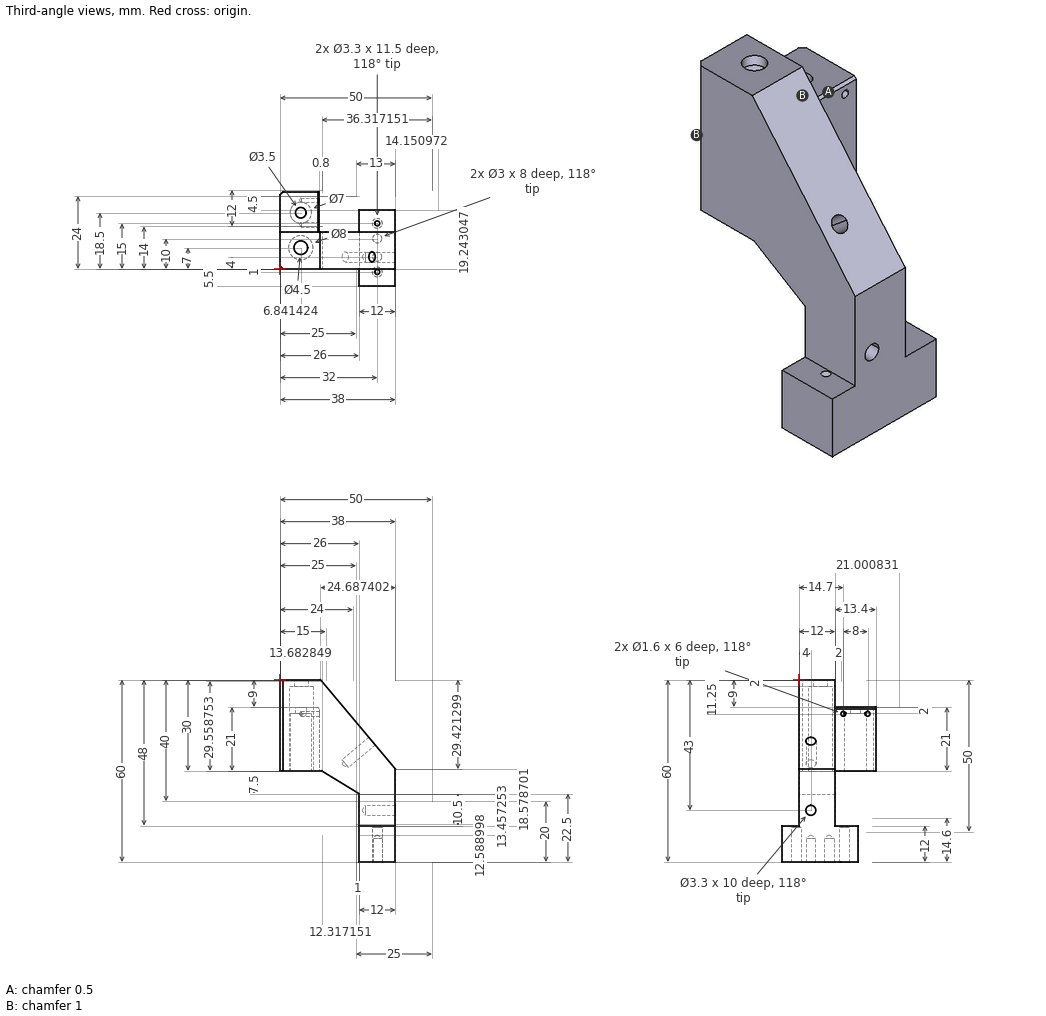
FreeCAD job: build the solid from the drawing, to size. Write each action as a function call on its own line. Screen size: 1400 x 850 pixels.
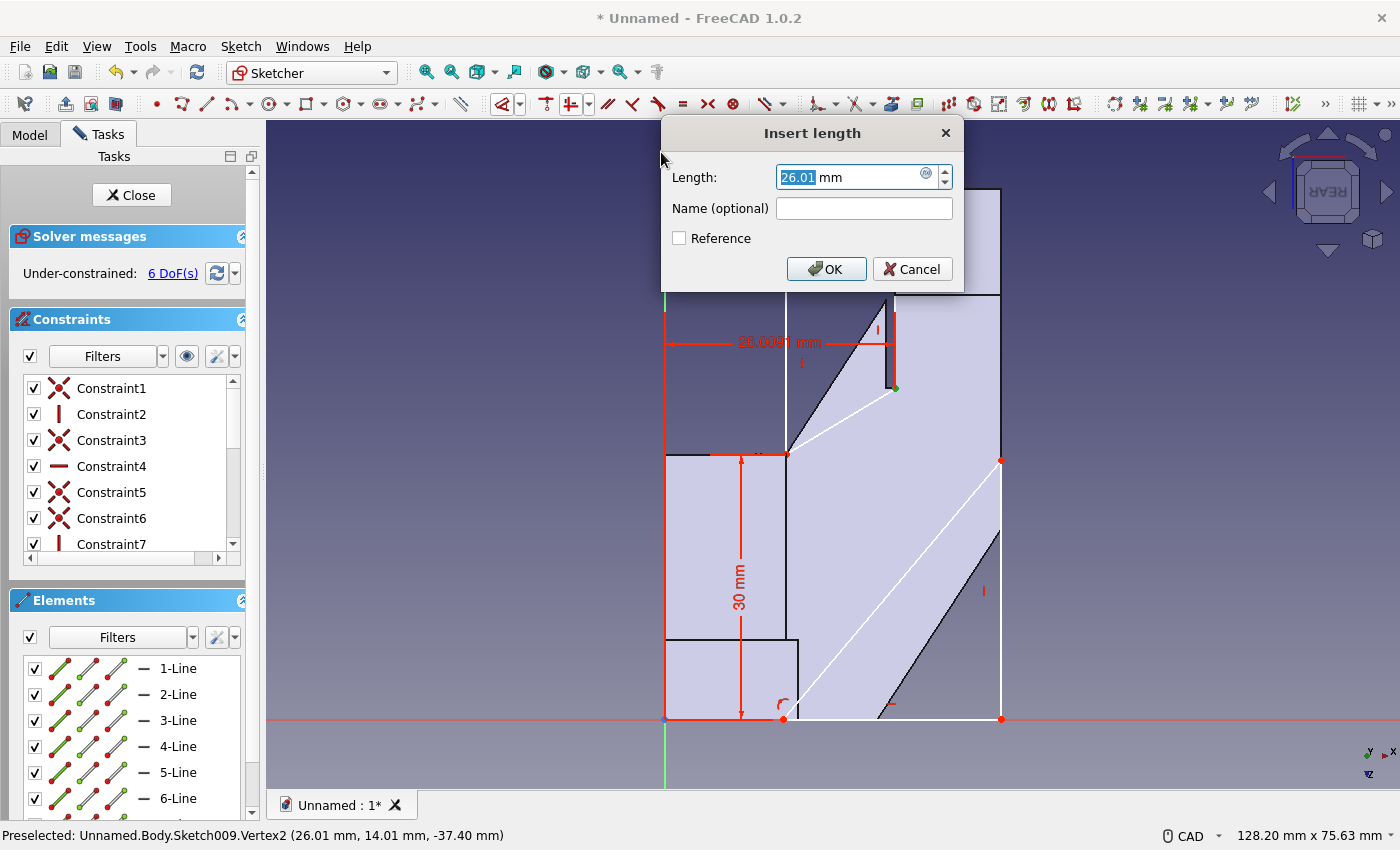
text(26)
key(Return)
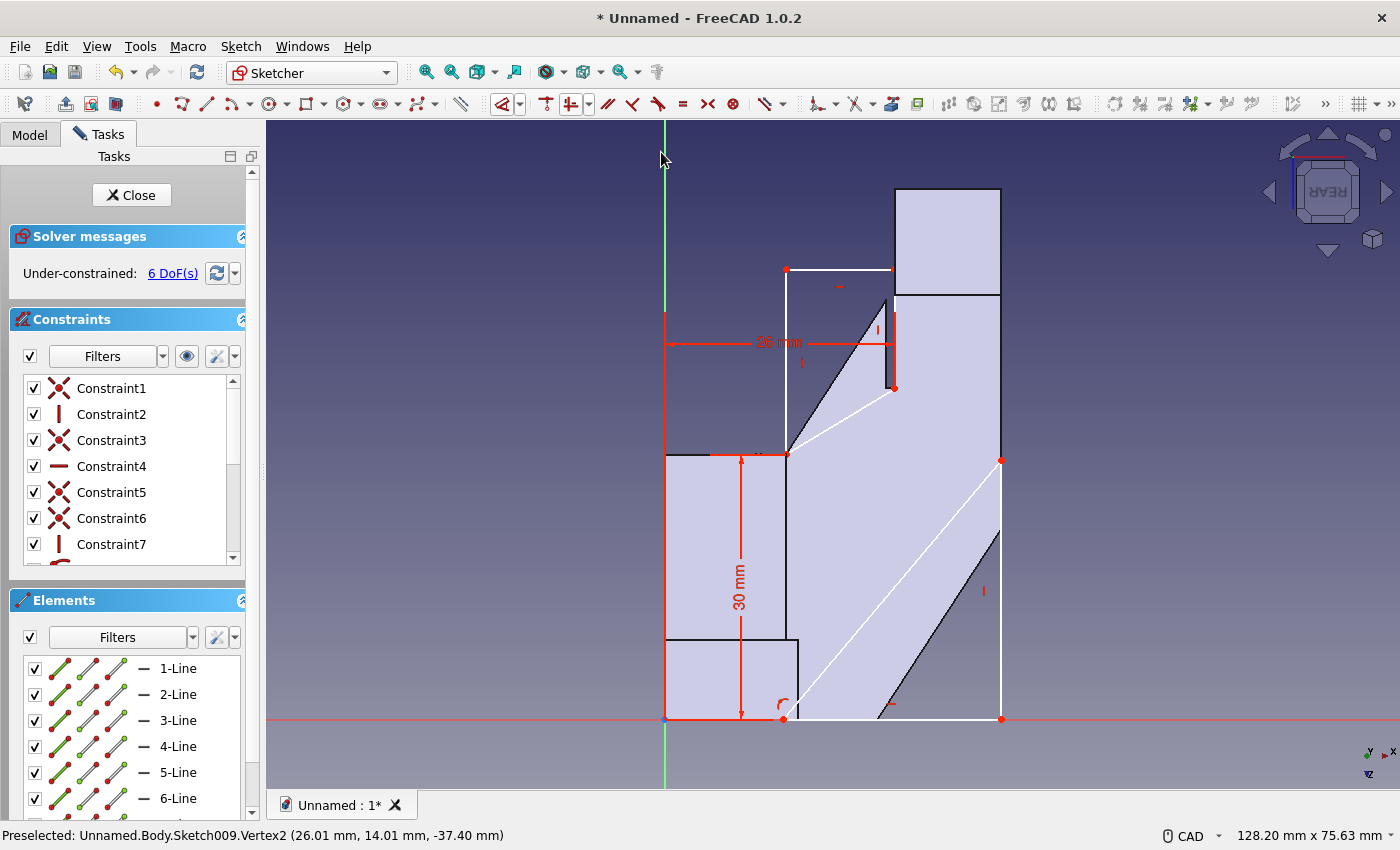
click(1001, 720)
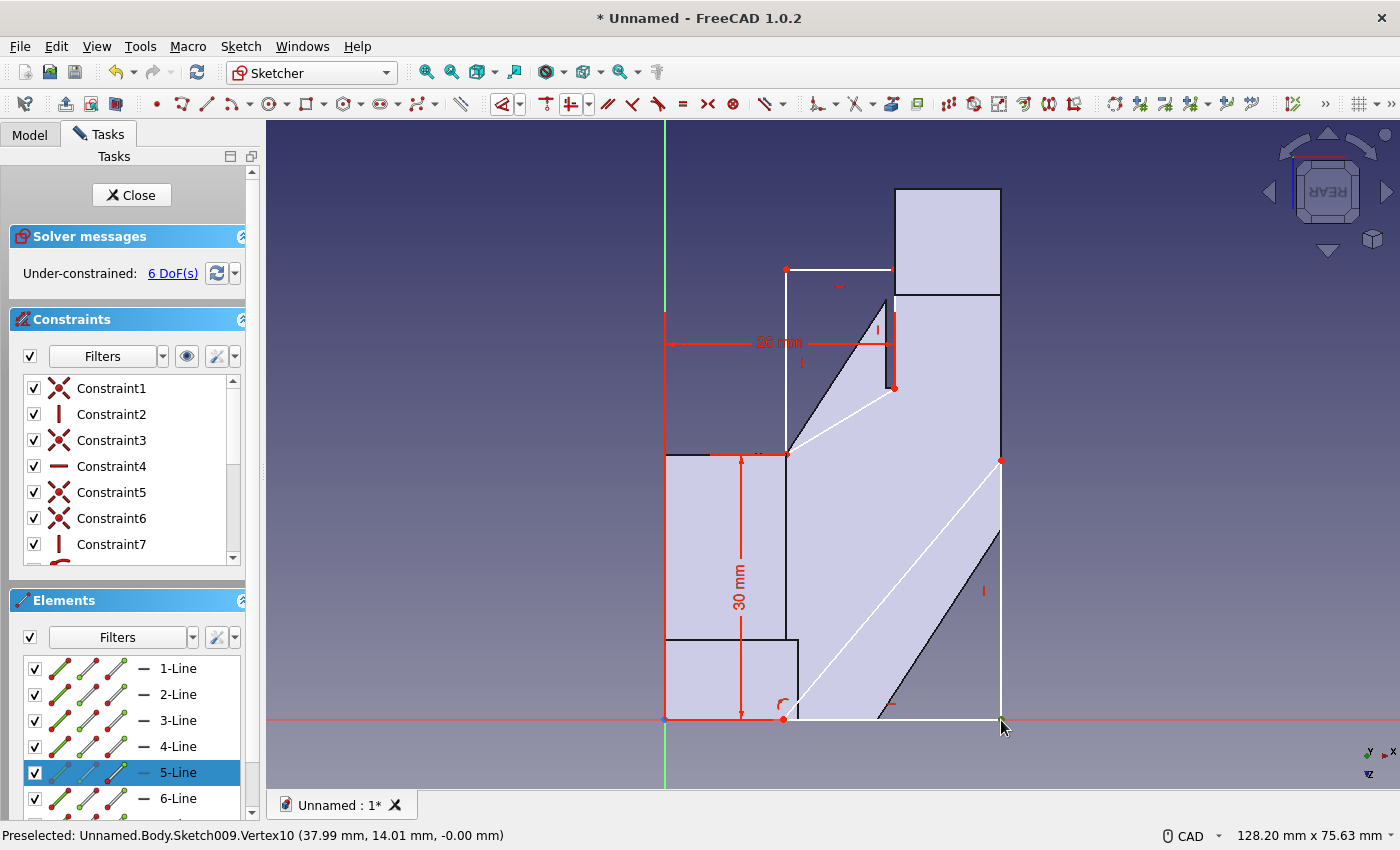
click(520, 104)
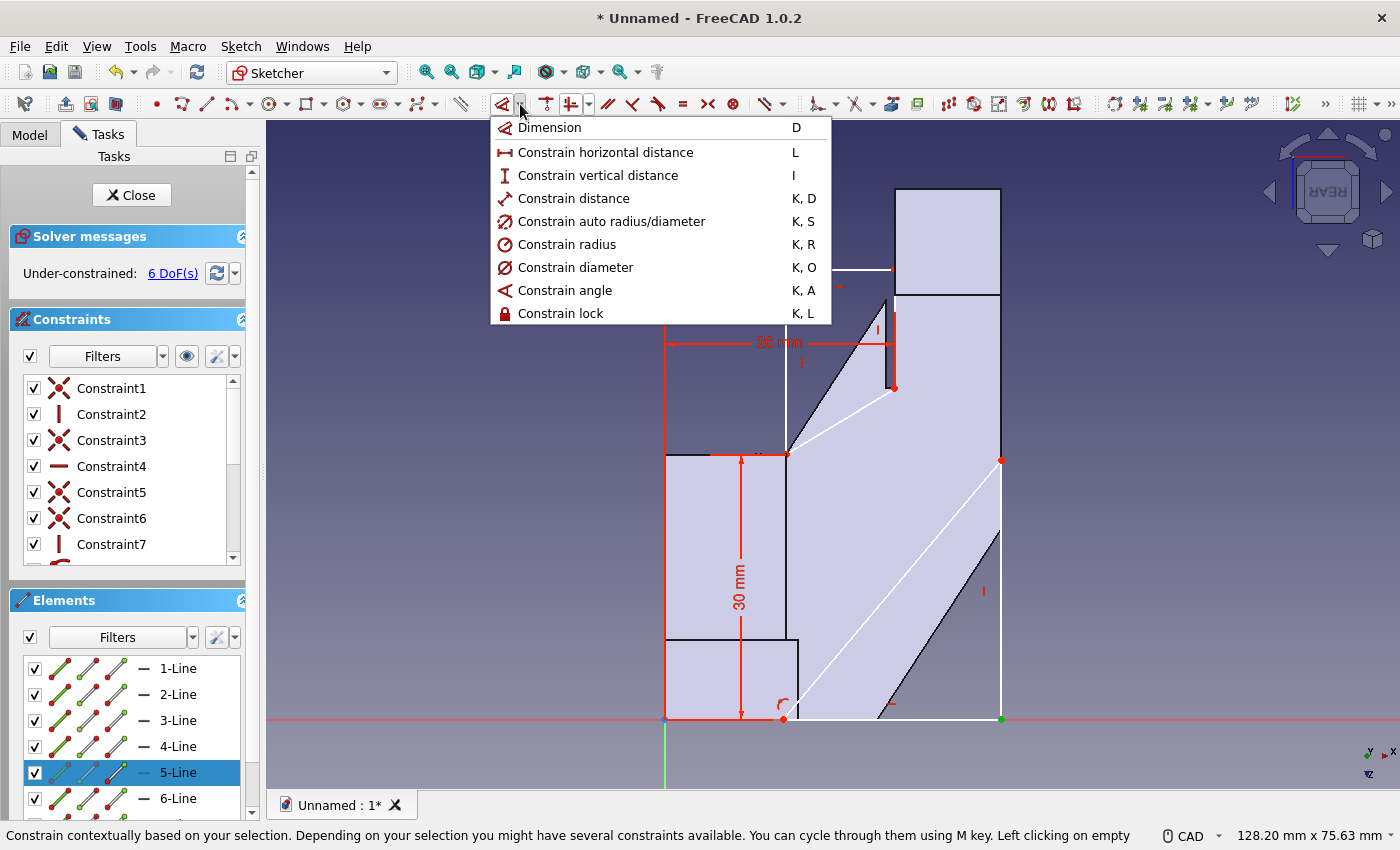
click(661, 152)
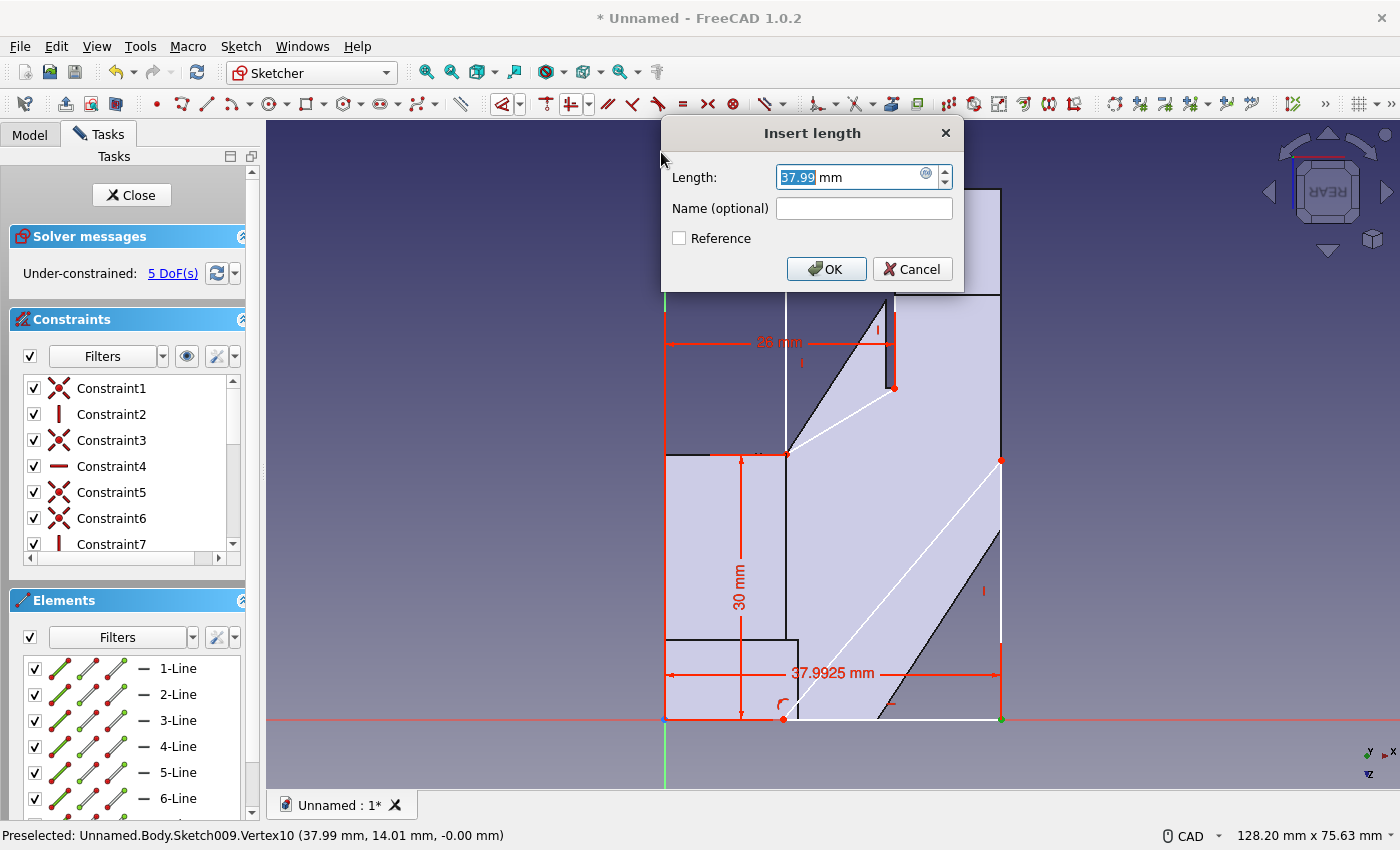
text(38)
key(Return)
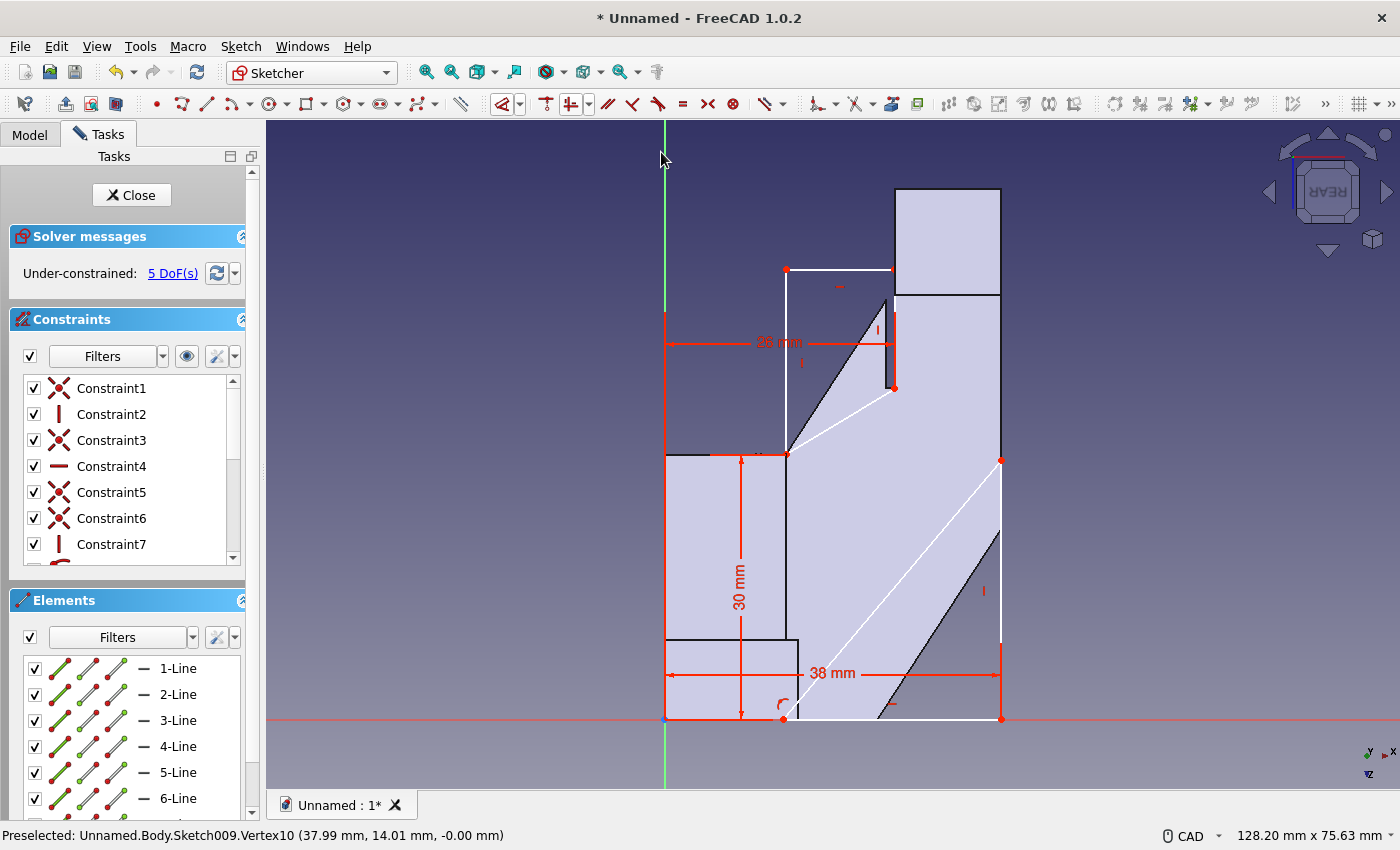
click(819, 435)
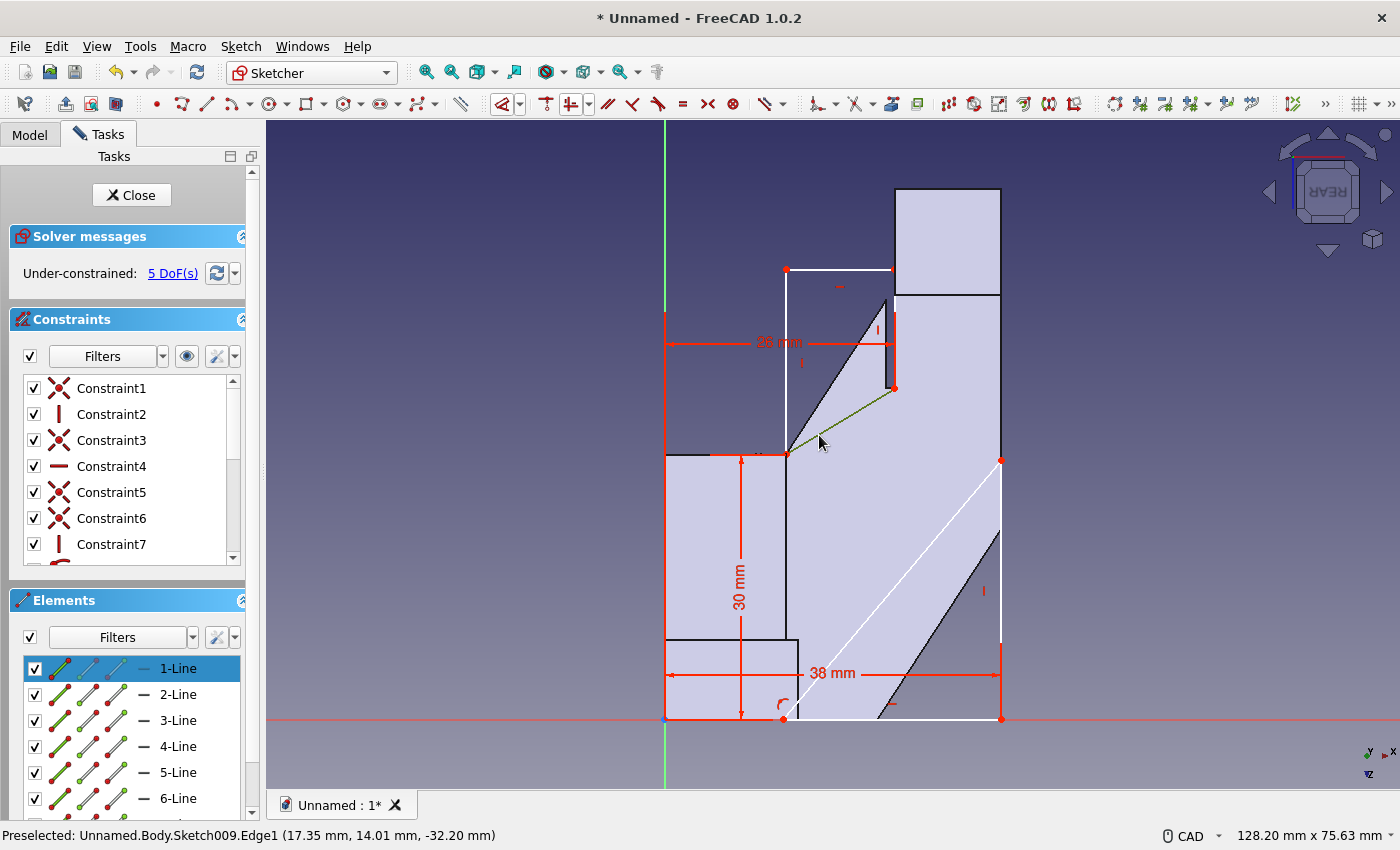
click(520, 104)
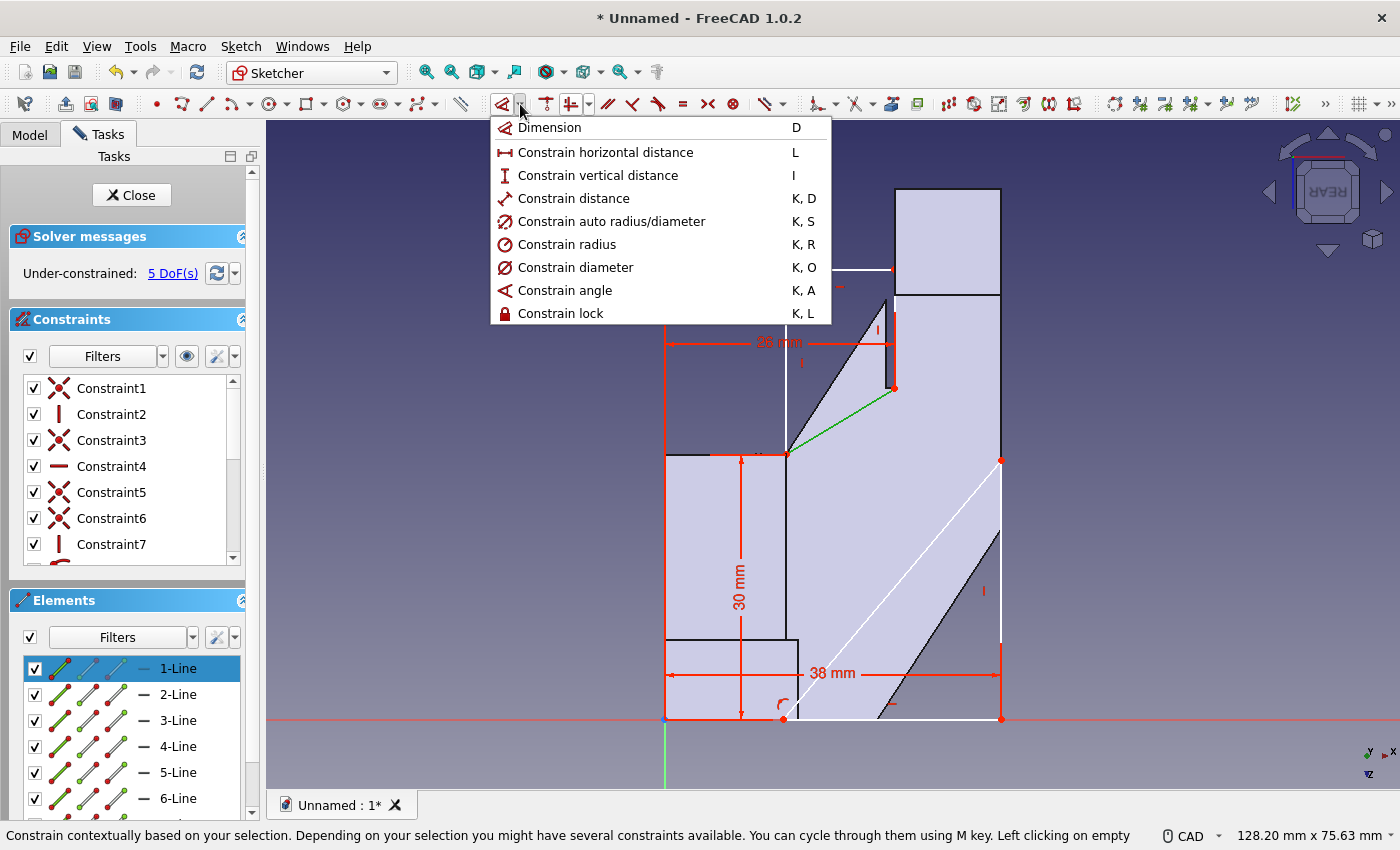
click(661, 176)